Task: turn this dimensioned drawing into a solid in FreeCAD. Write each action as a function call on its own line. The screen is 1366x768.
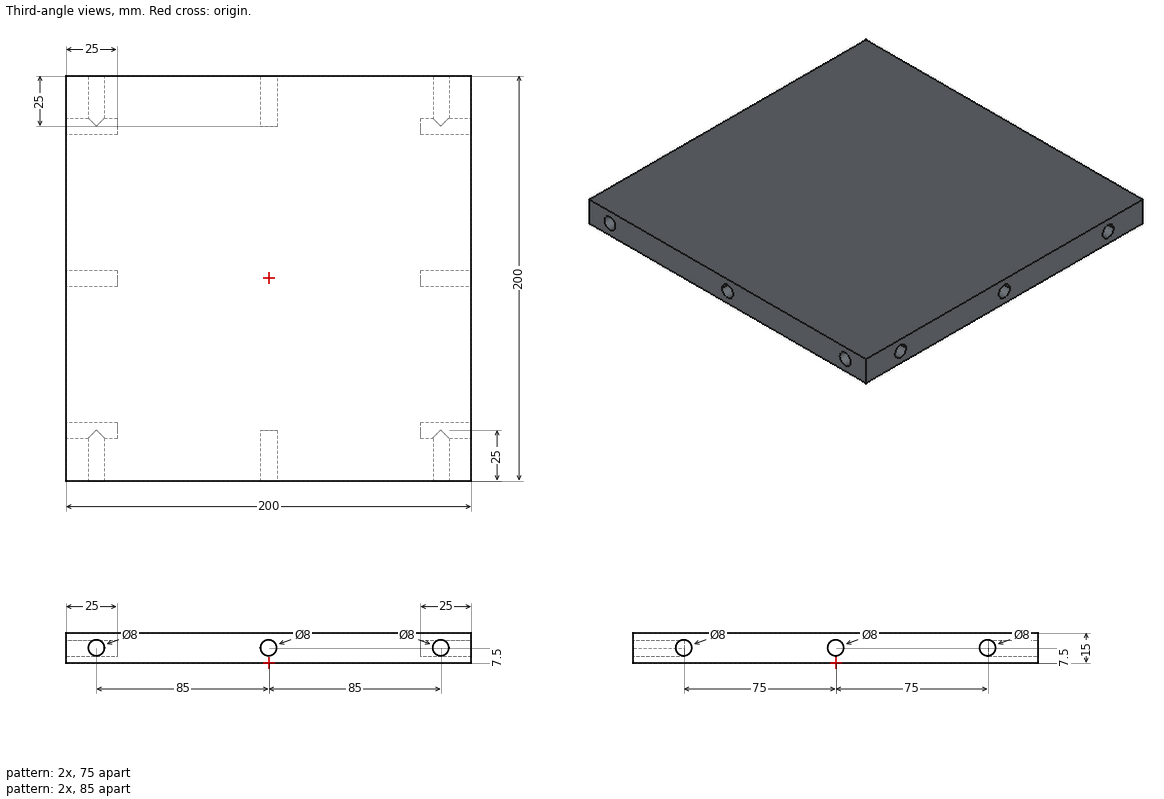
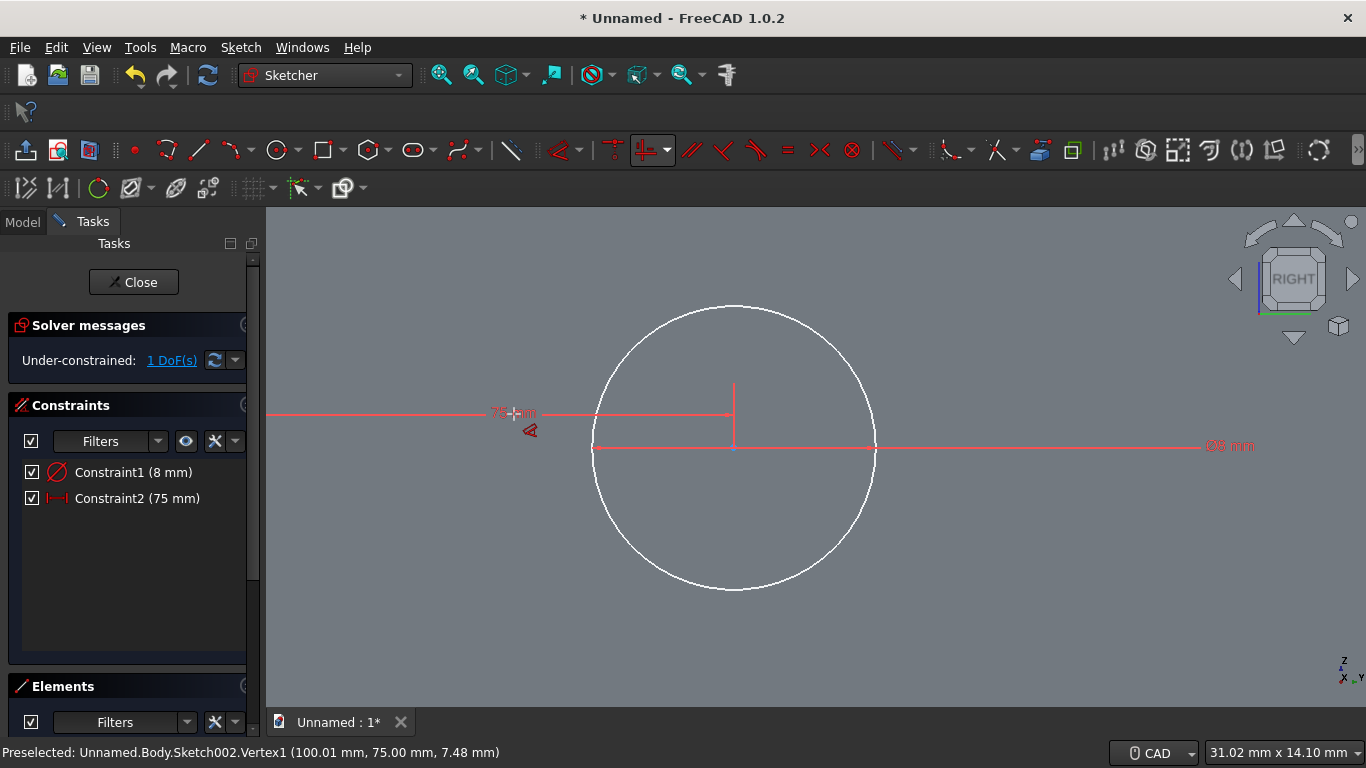
click(734, 448)
click(768, 563)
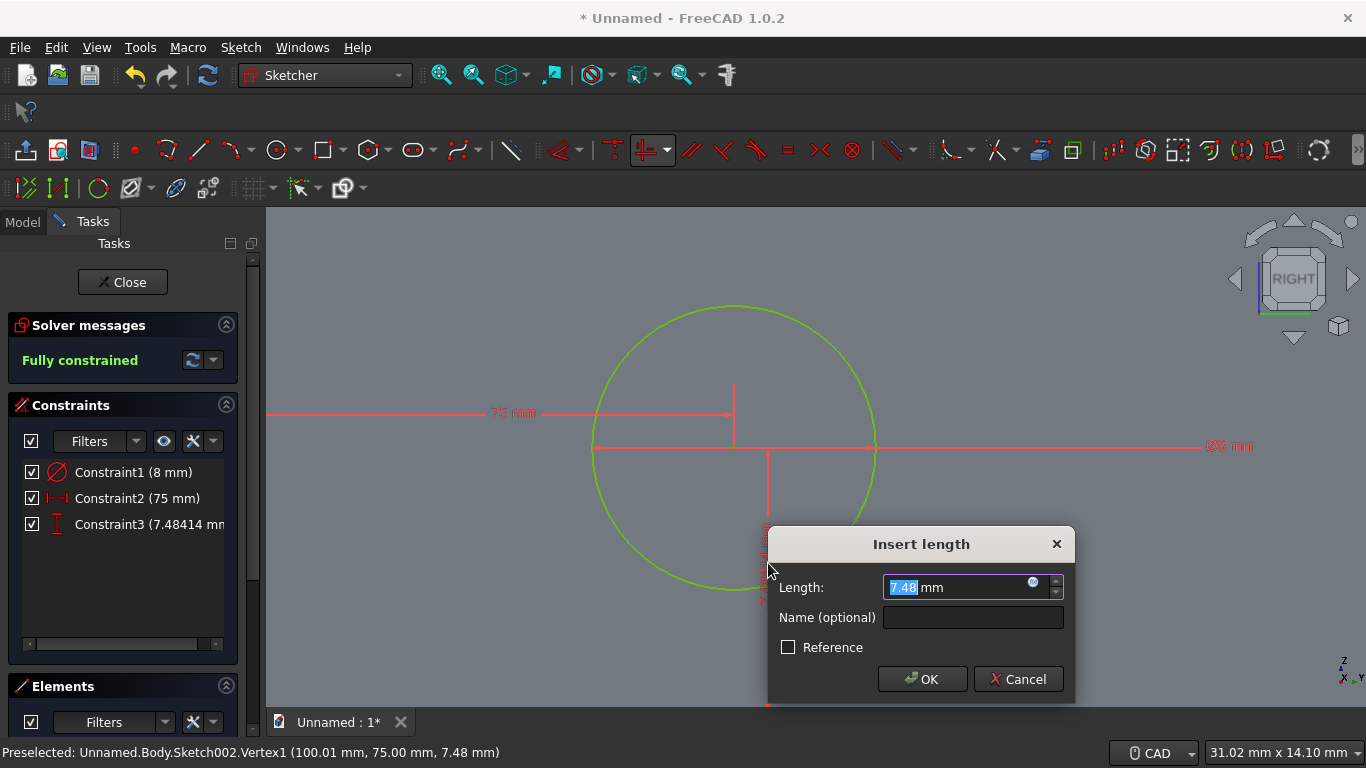
text(7.5)
key(Return)
key(Escape)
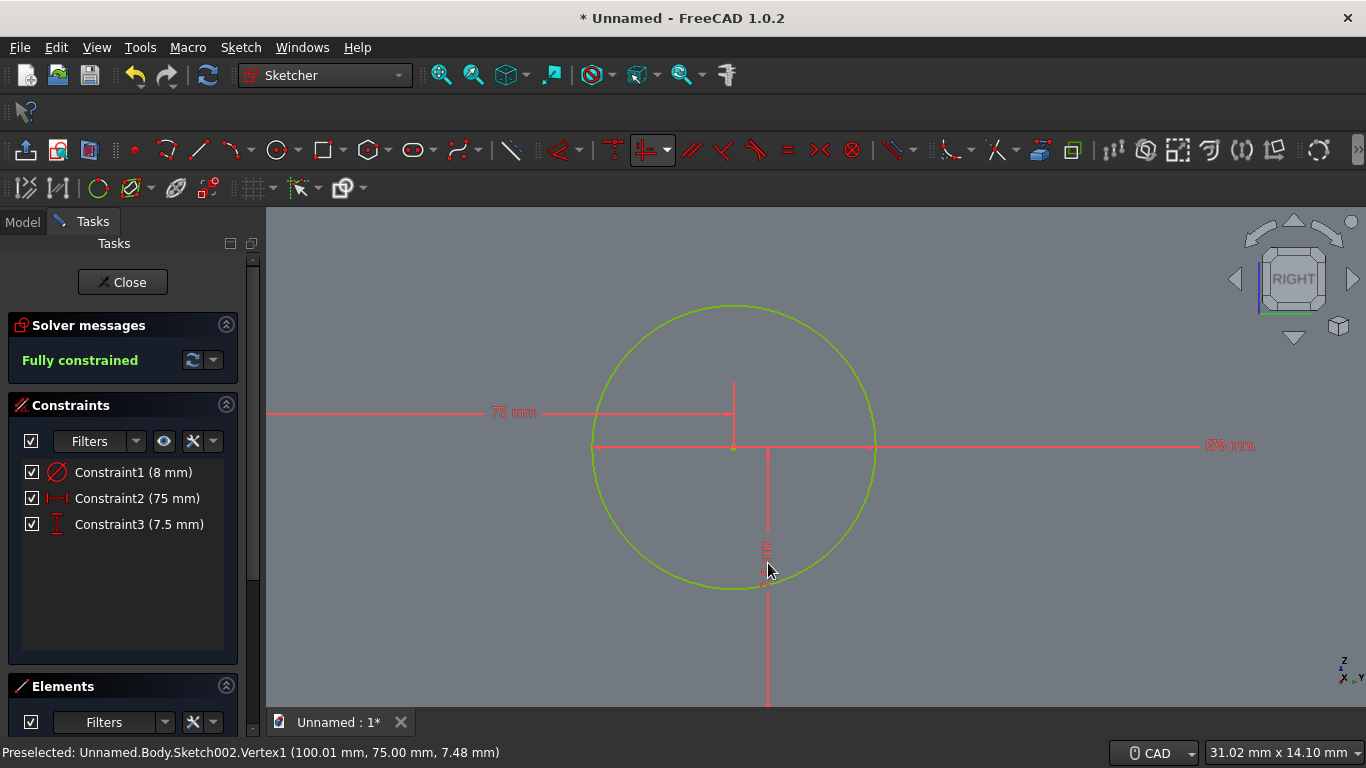
click(123, 282)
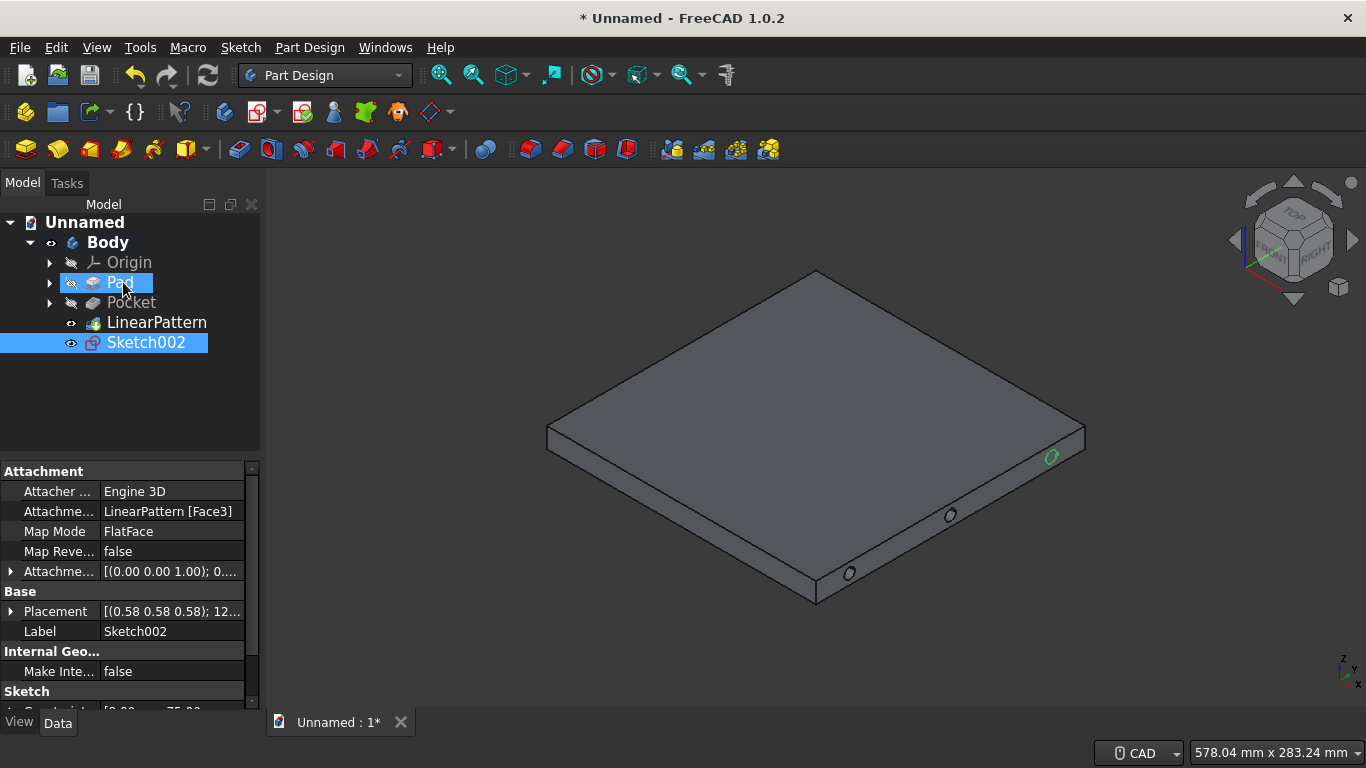
click(240, 150)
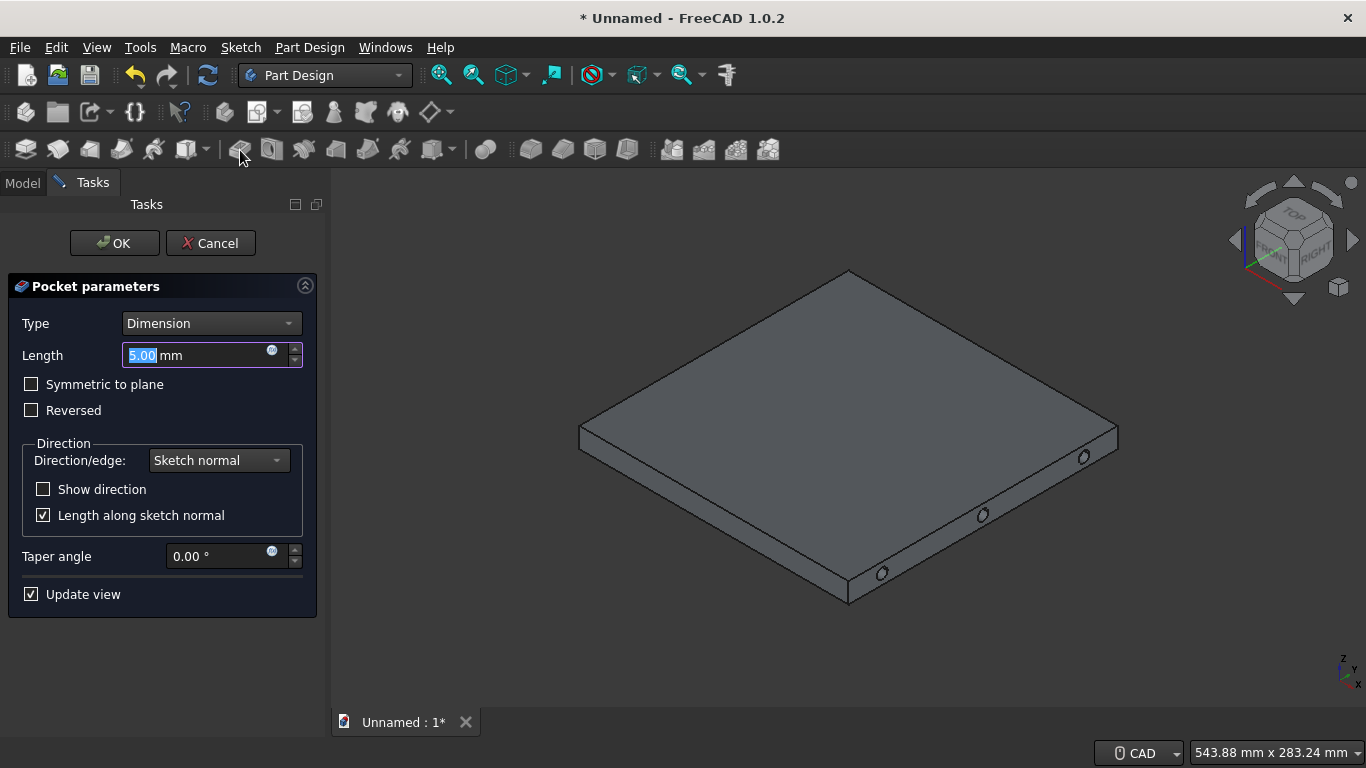
text(25)
key(Tab)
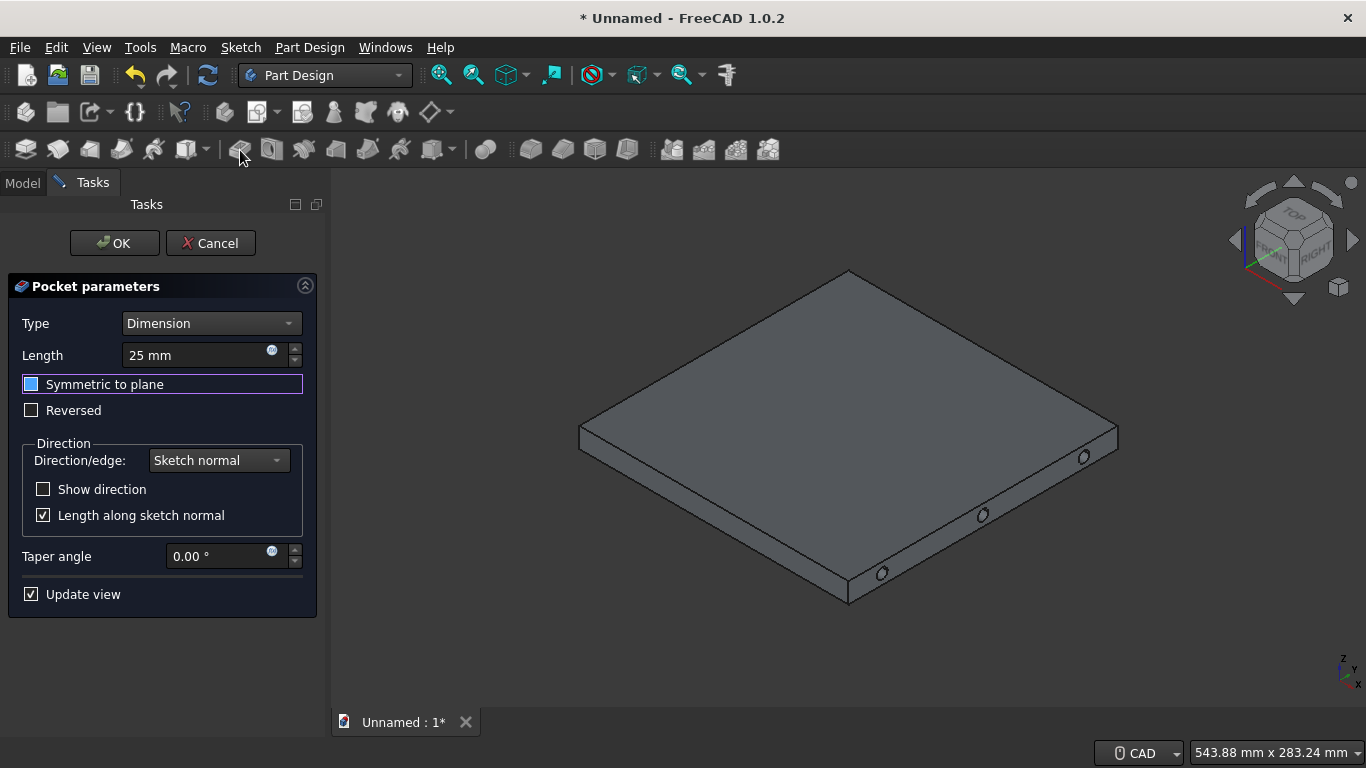
click(115, 243)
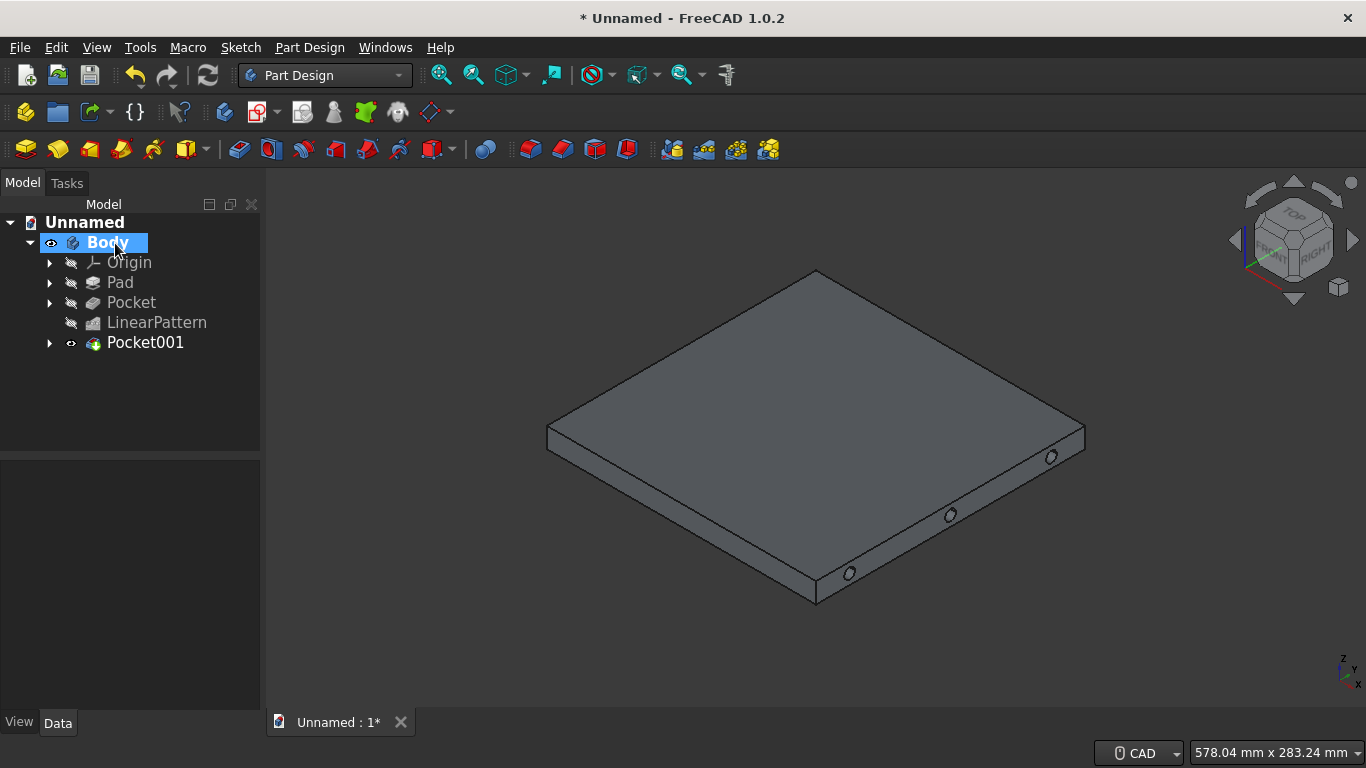
click(116, 303)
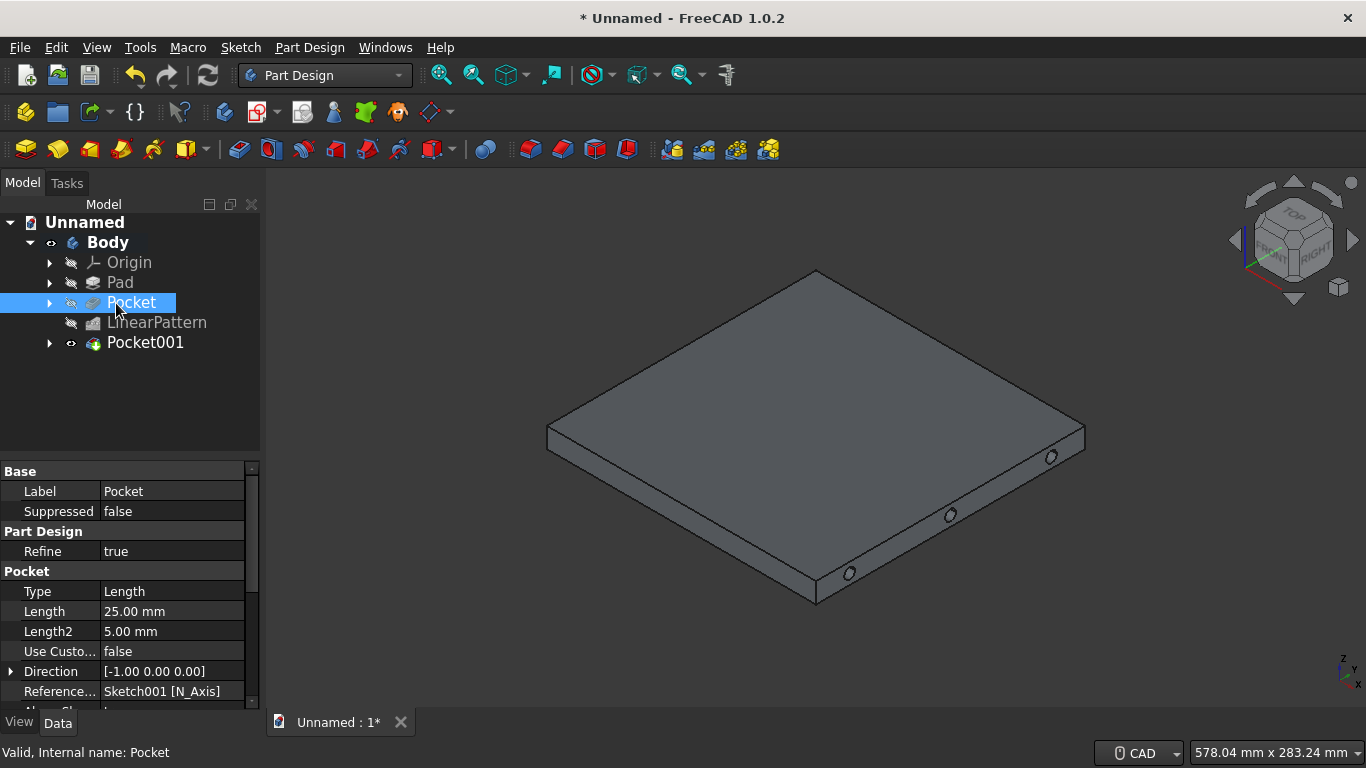
click(672, 150)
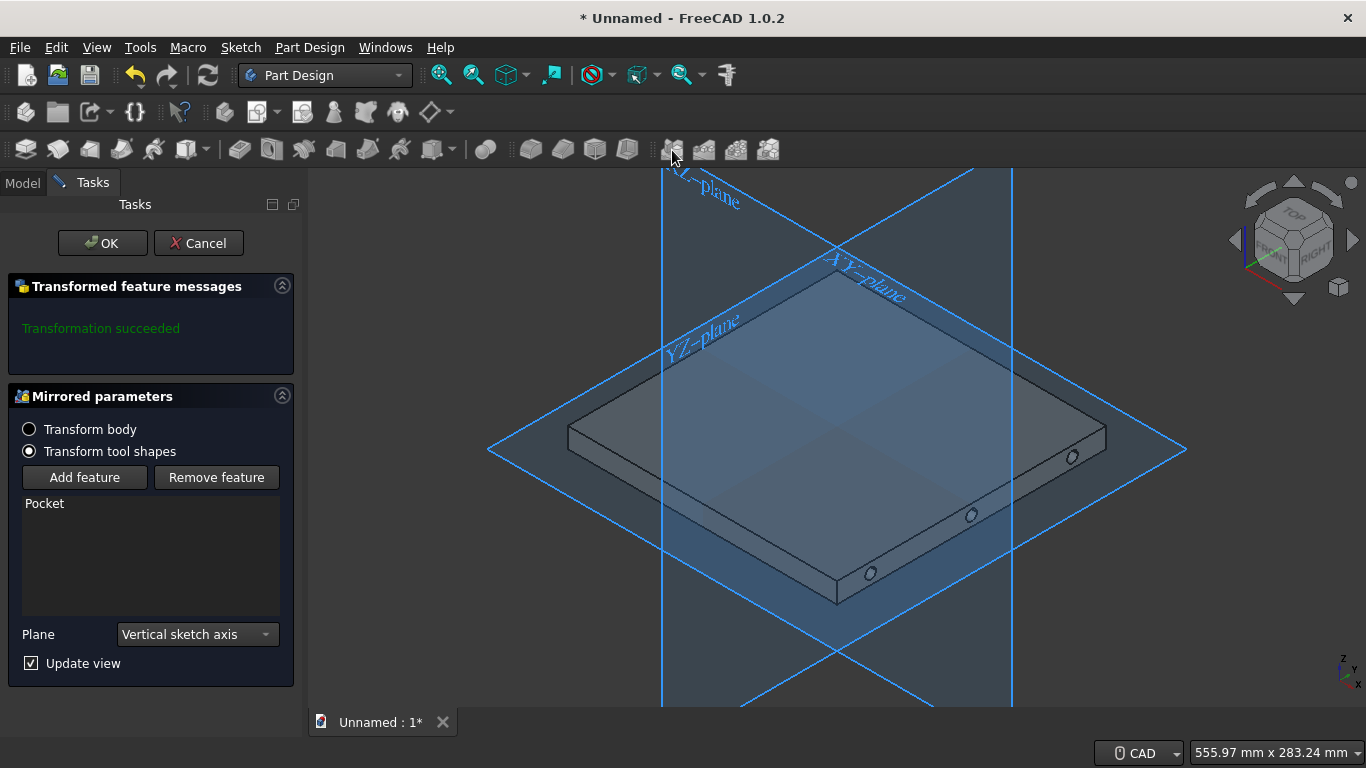
click(198, 634)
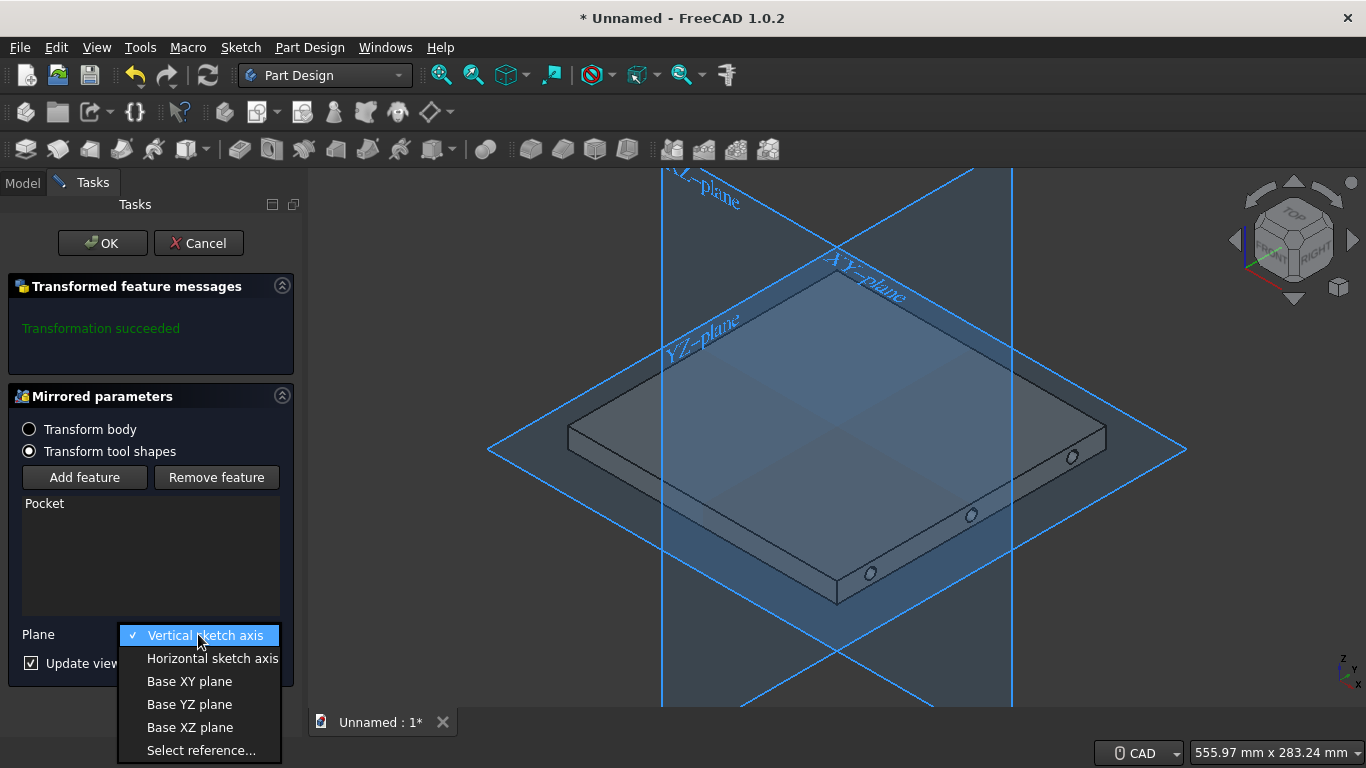
click(198, 704)